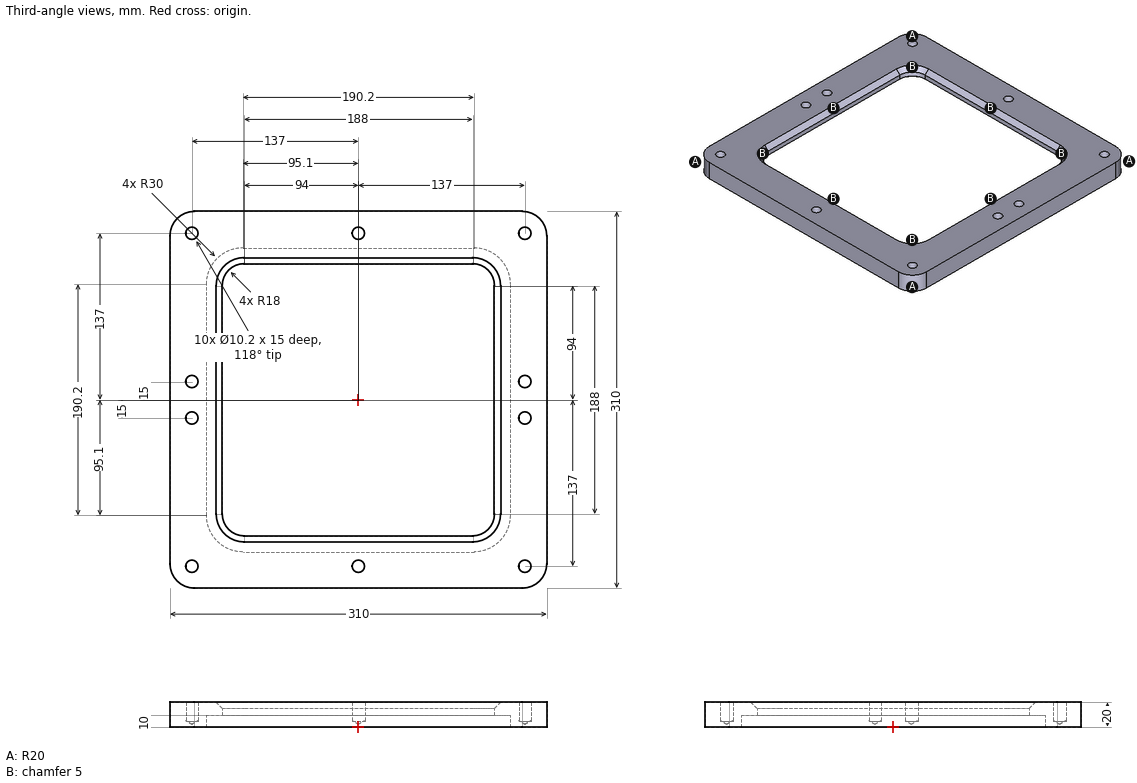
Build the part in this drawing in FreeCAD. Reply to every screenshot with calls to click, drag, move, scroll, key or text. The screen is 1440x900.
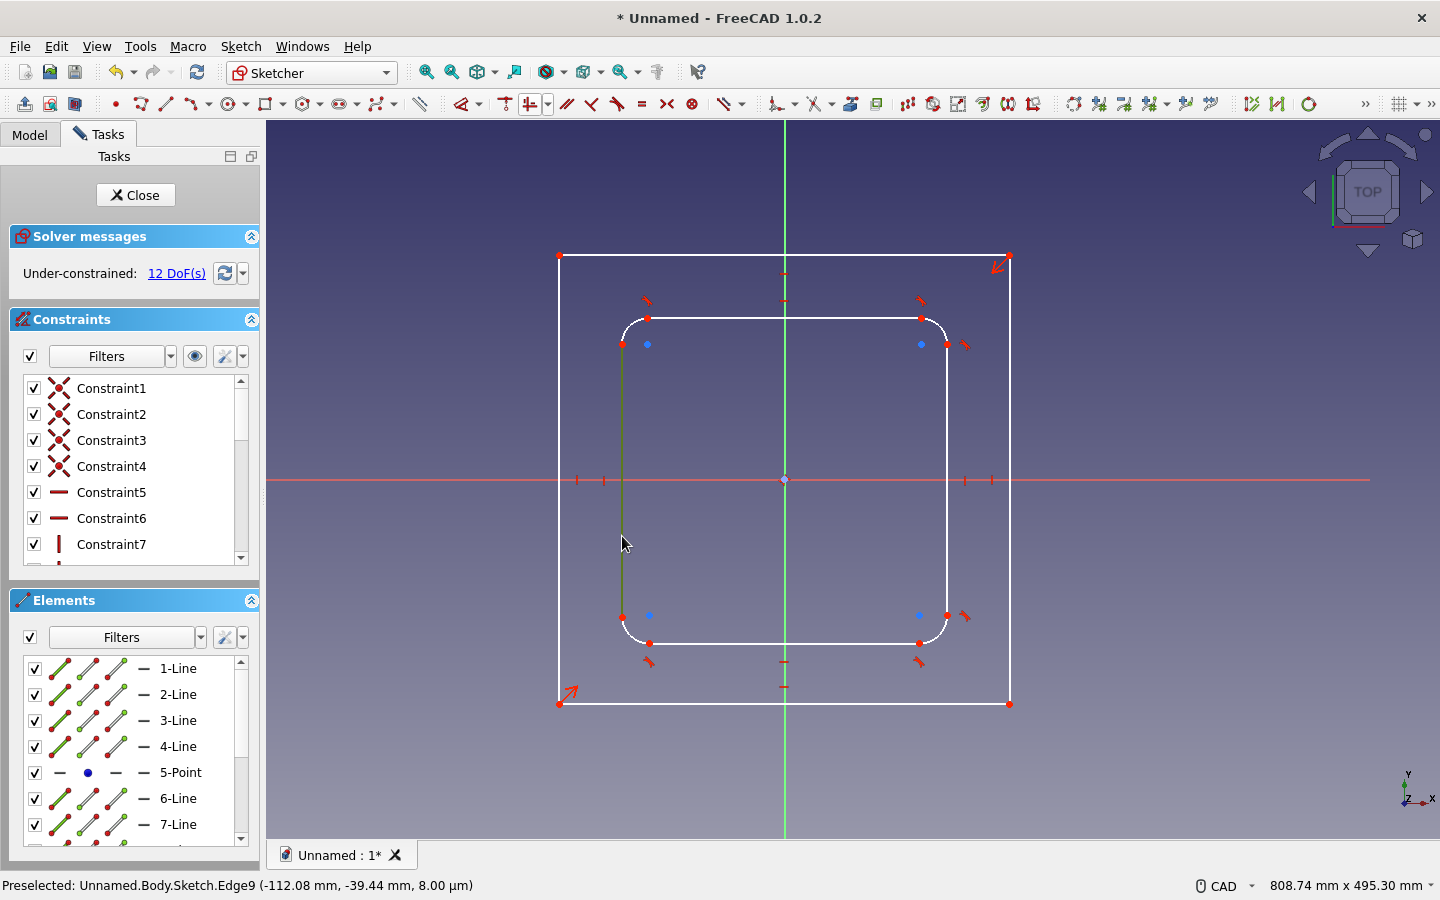
click(626, 629)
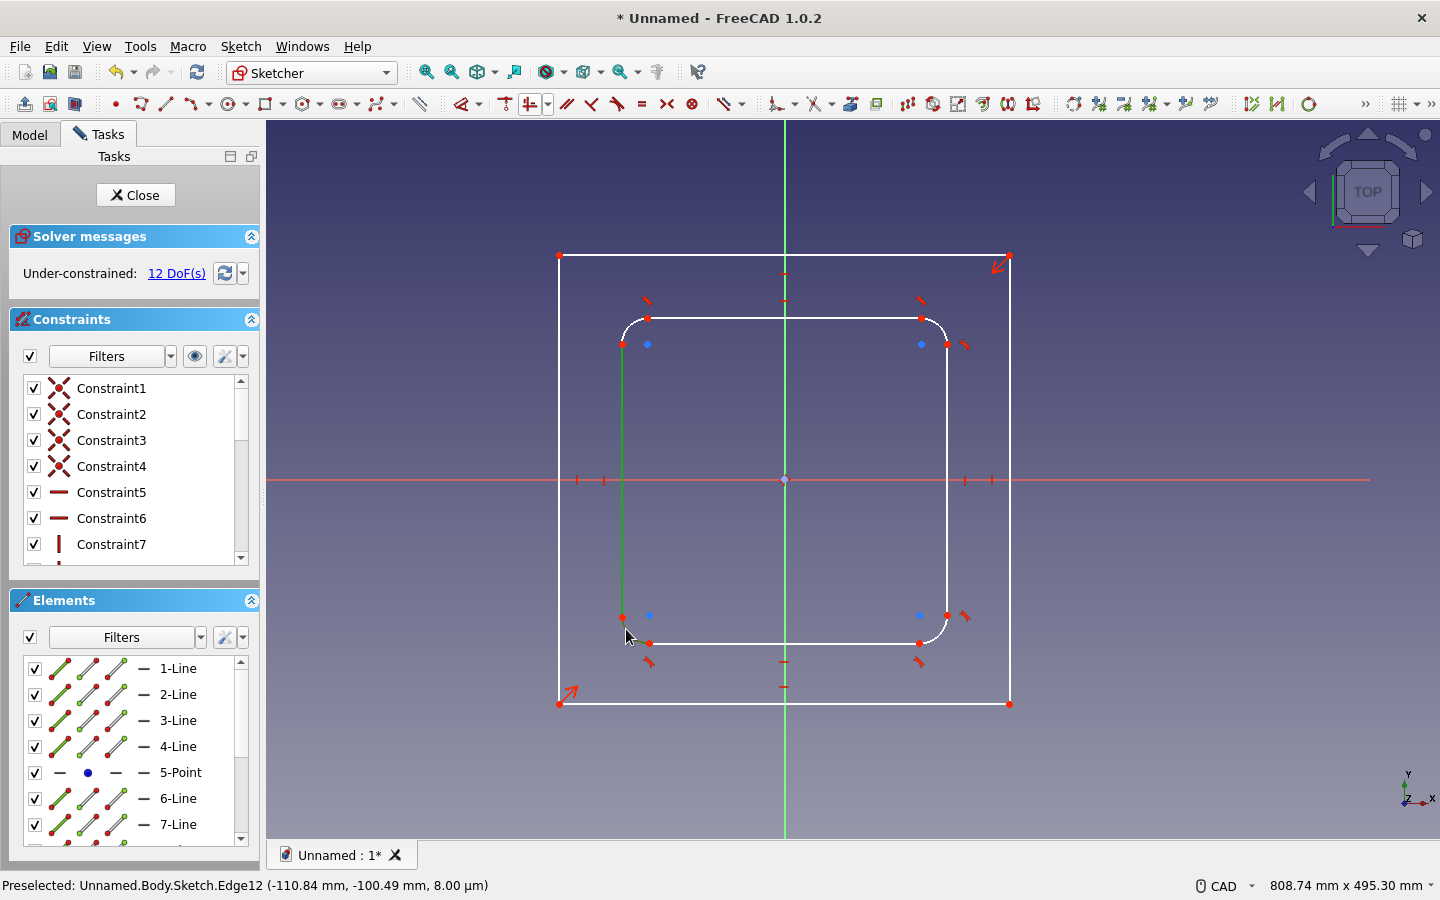
click(617, 104)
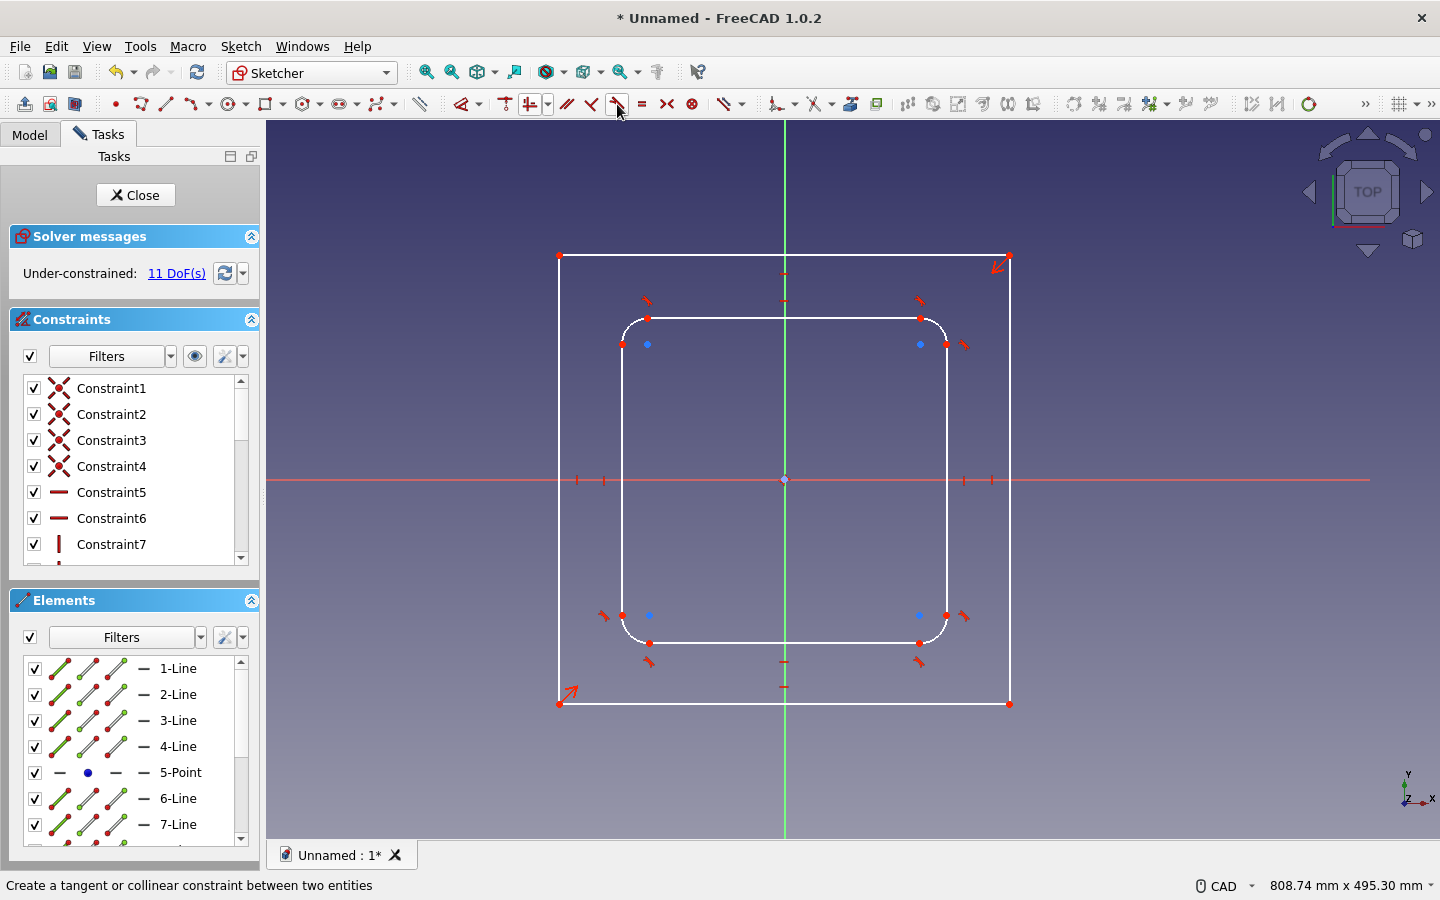
click(622, 534)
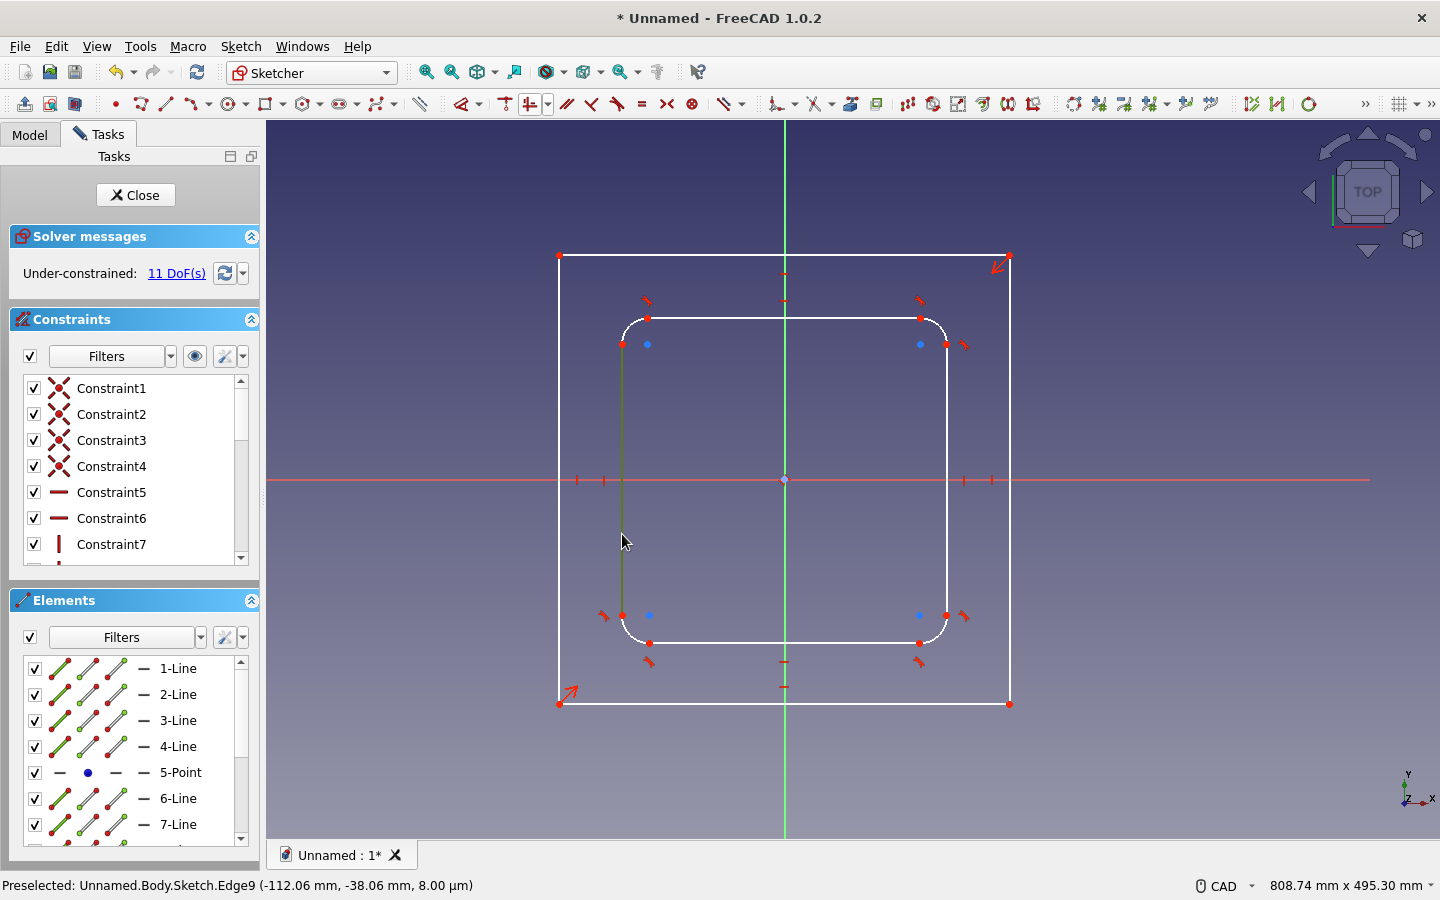
click(636, 321)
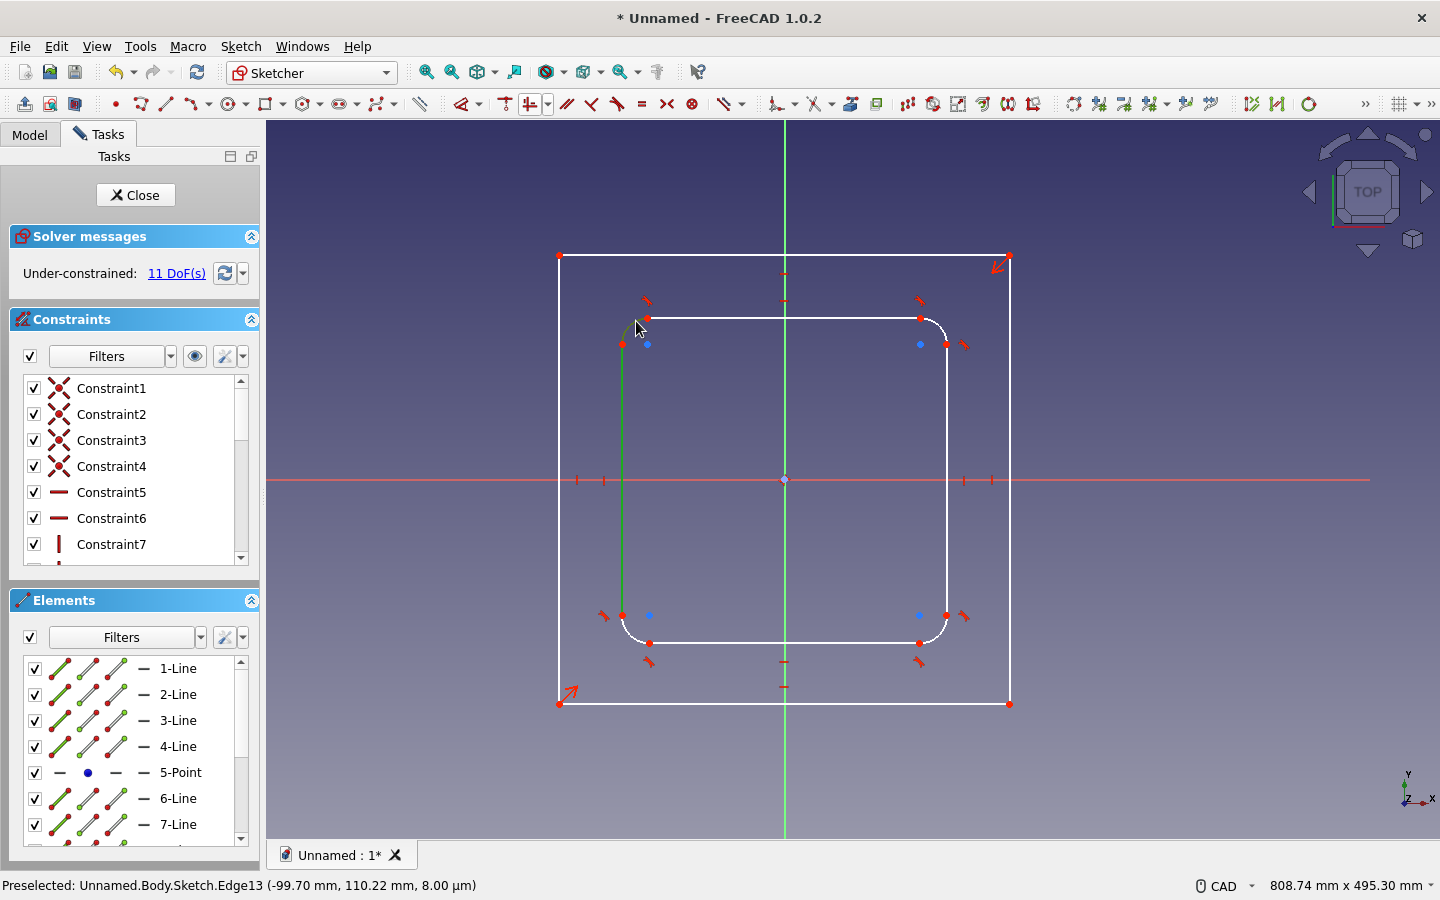
click(617, 104)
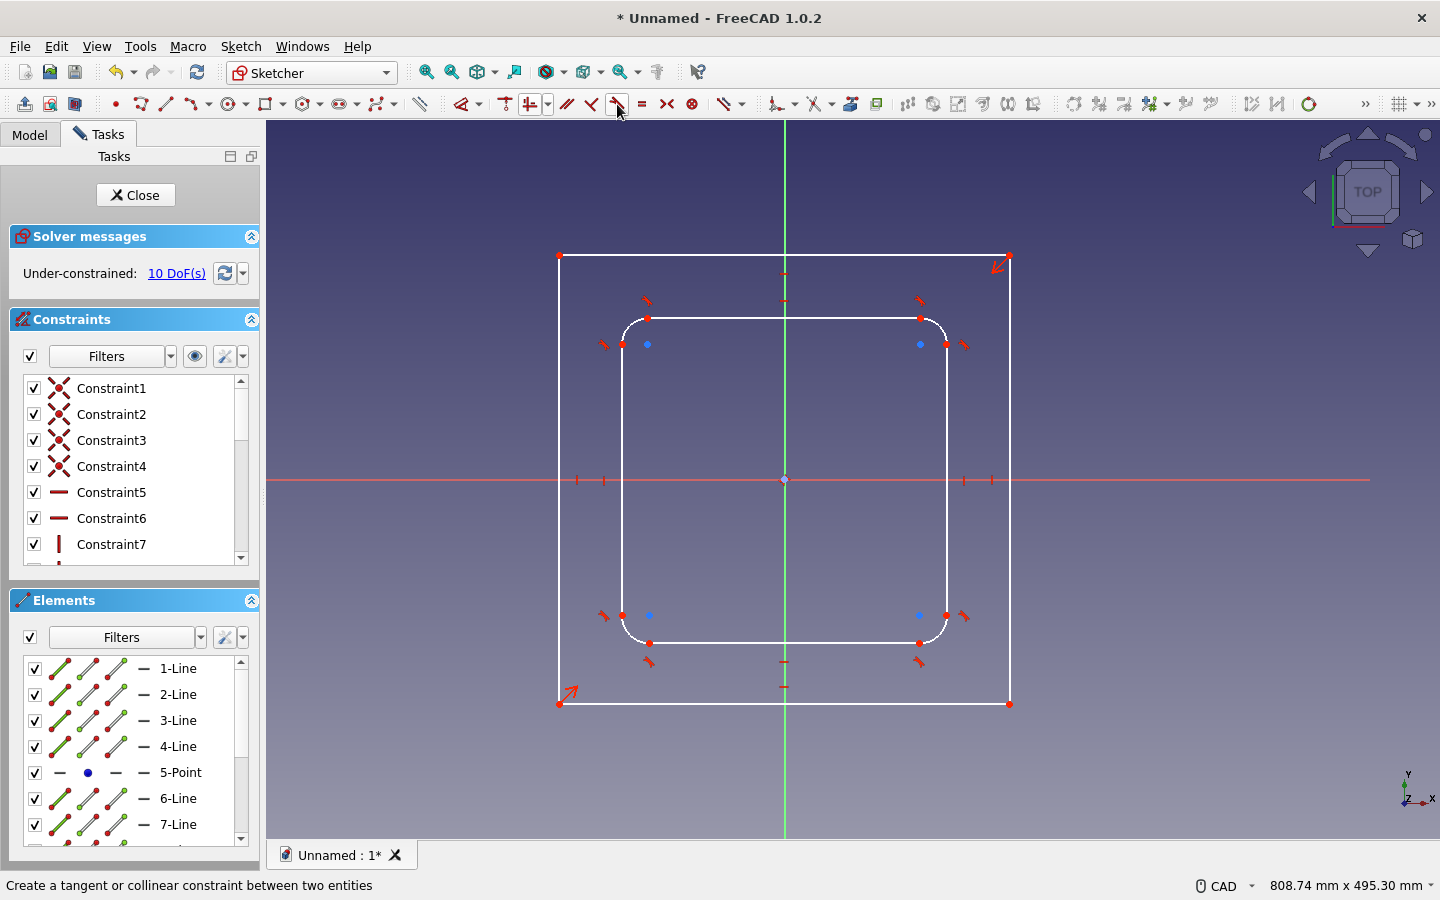
click(944, 333)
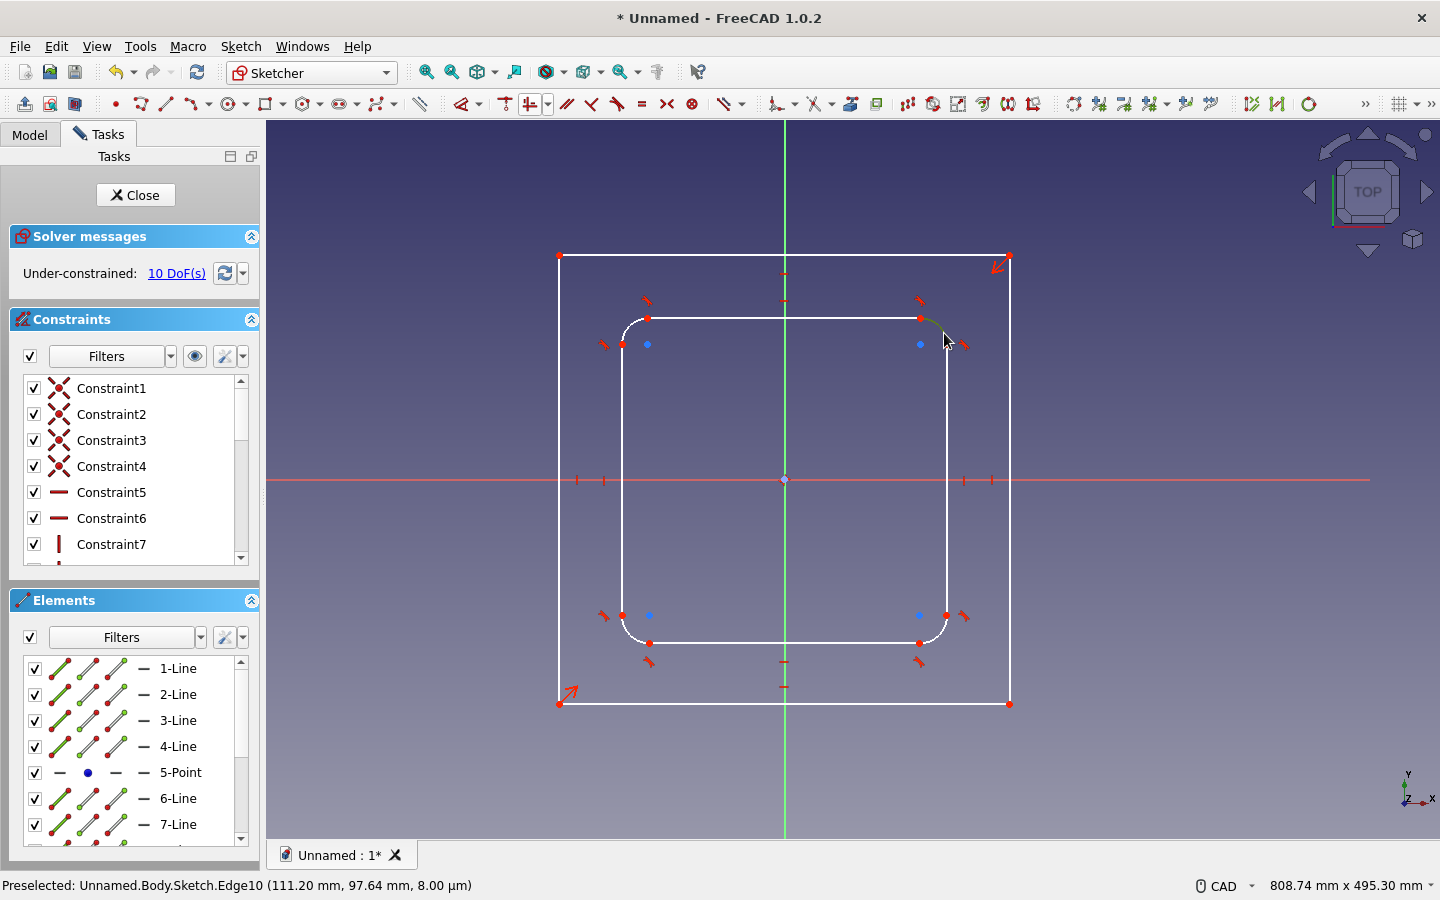
click(932, 640)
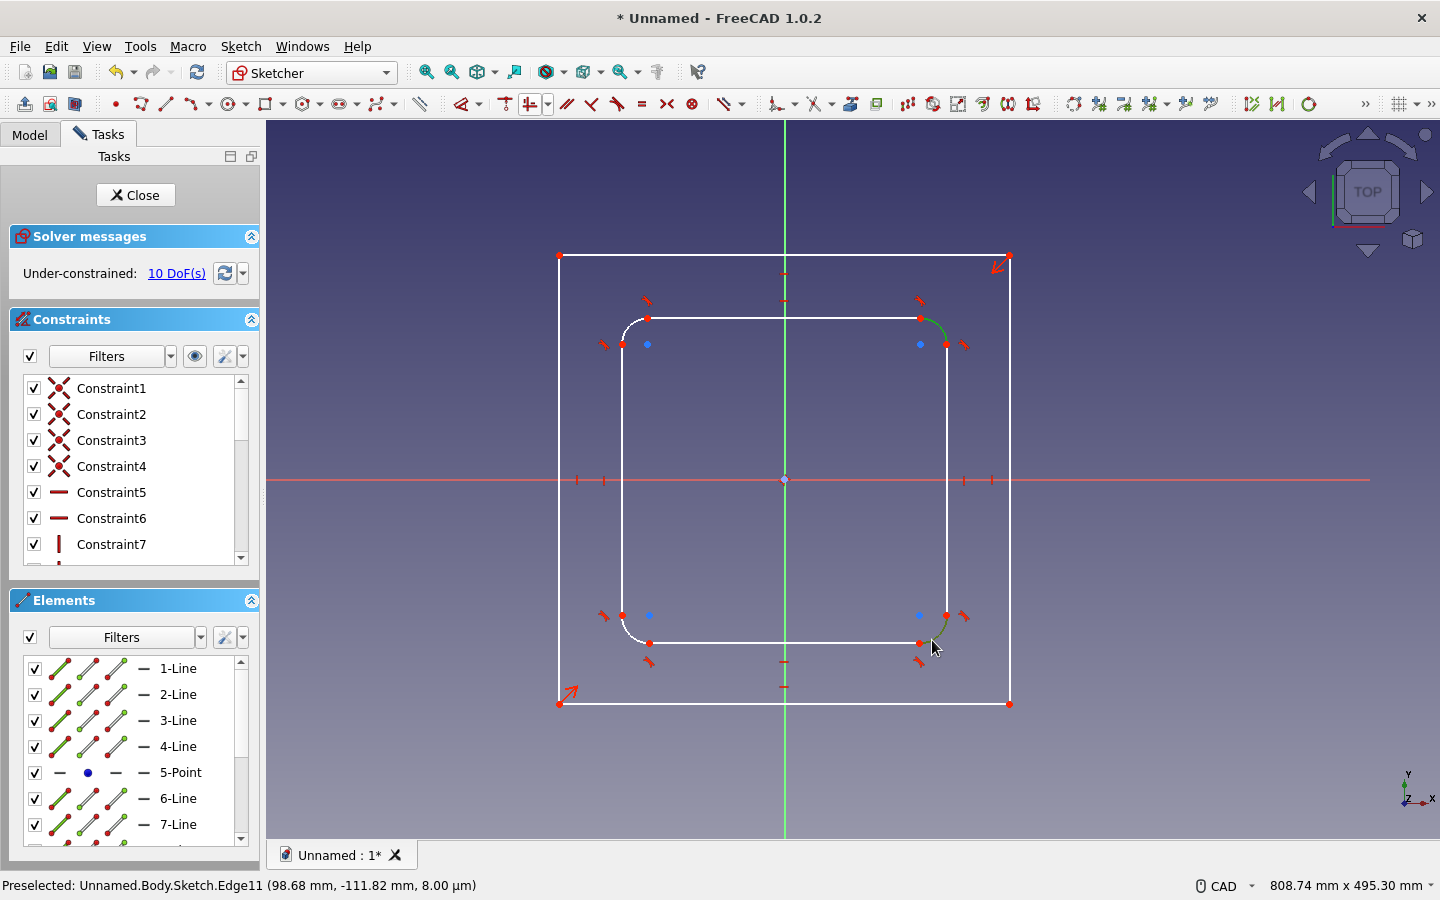
click(625, 628)